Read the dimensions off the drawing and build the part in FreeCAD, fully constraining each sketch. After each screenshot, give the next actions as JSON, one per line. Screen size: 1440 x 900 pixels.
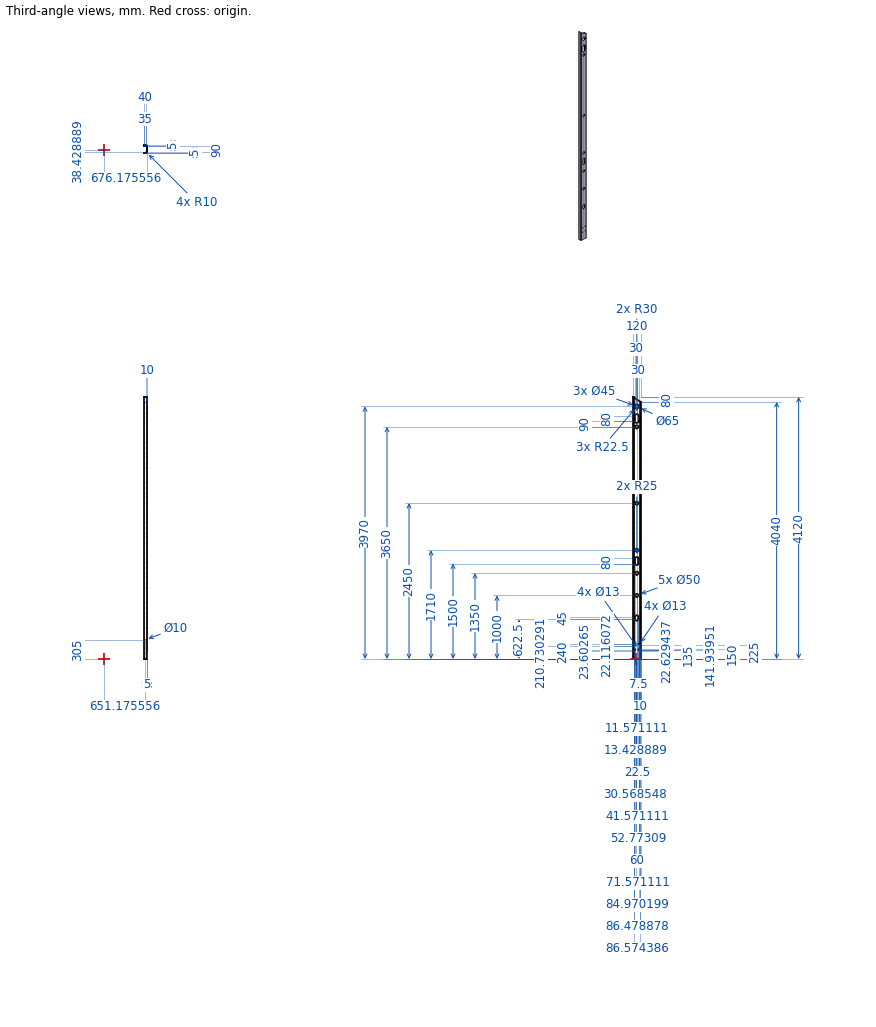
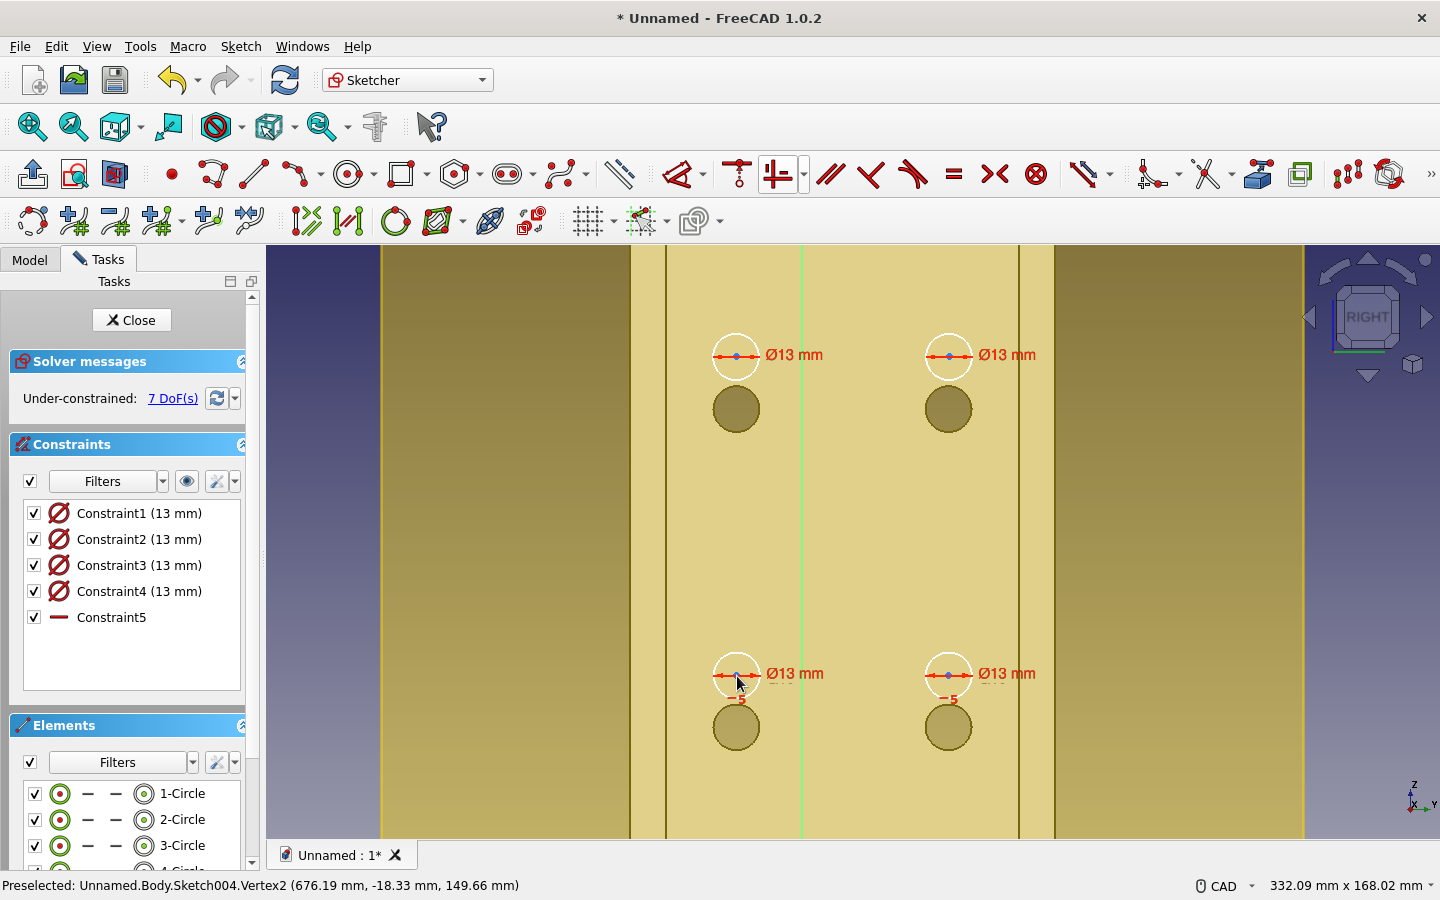
{"action": "left_click", "coordinate": [737, 676]}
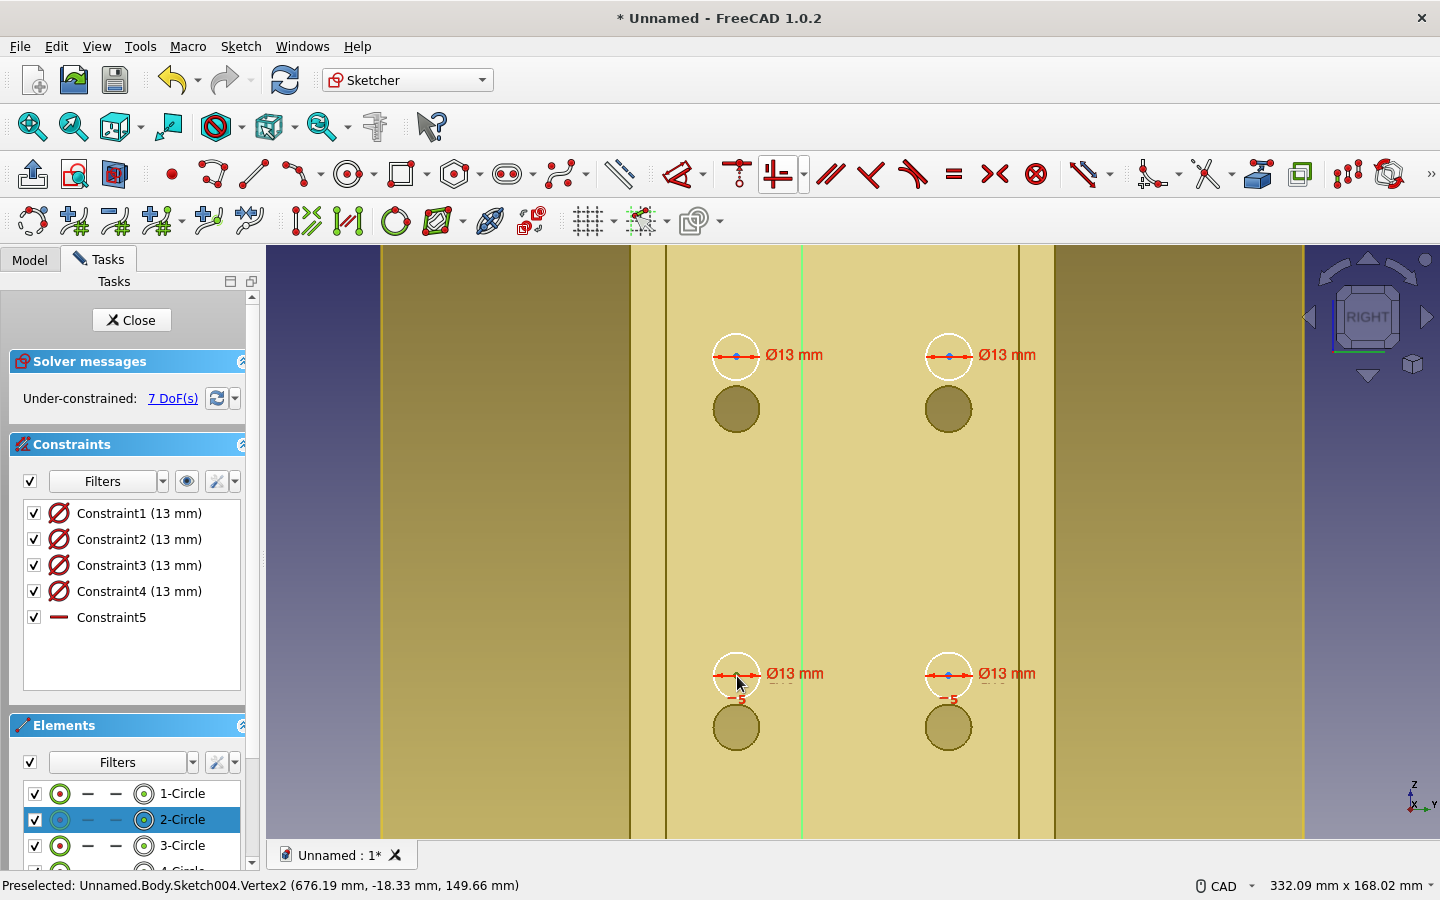
{"action": "left_click", "coordinate": [736, 357]}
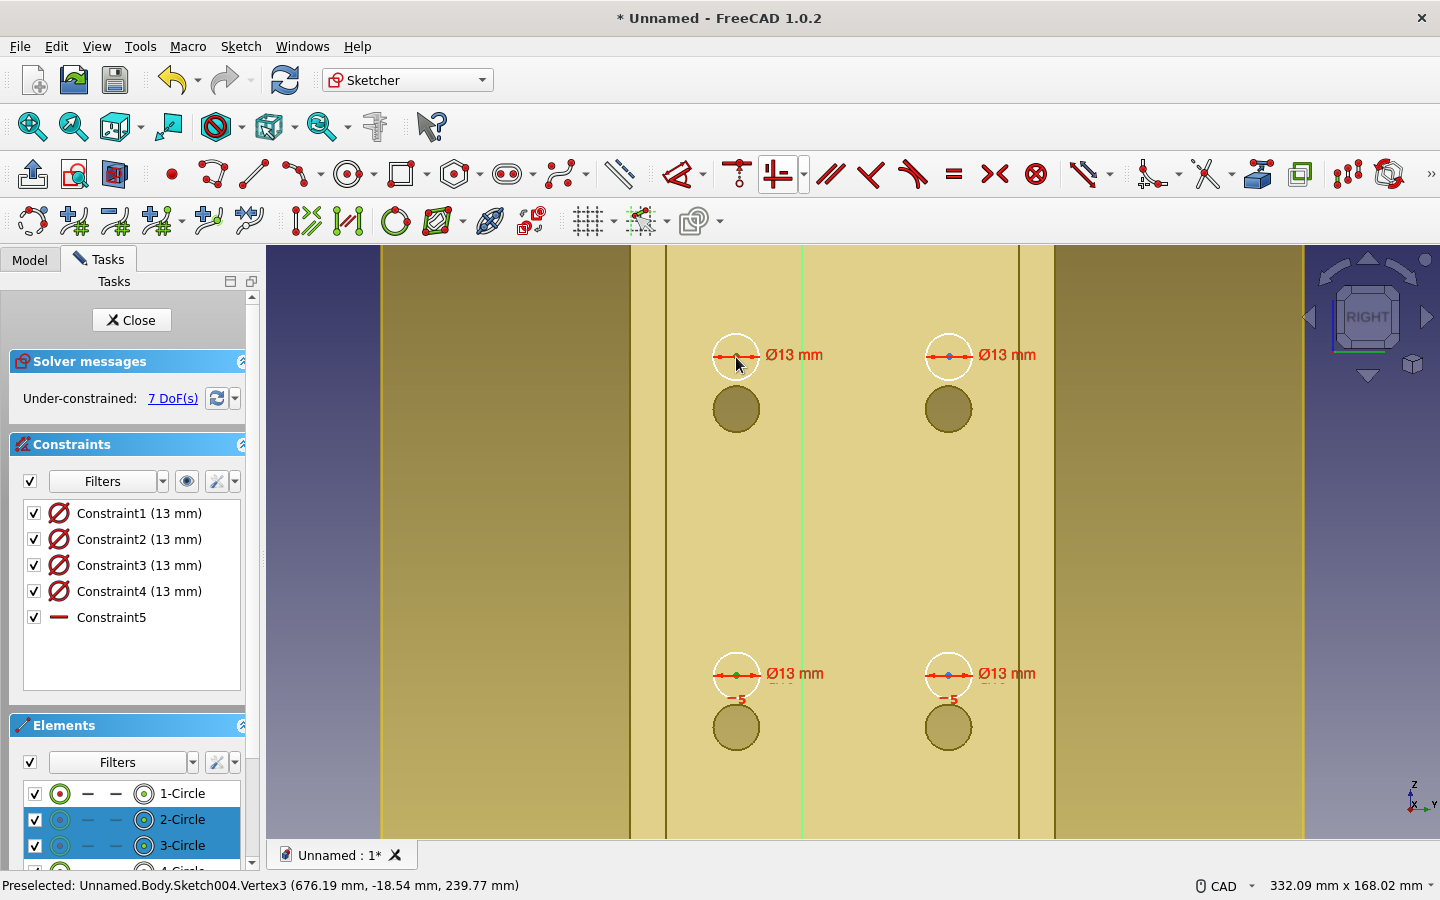
{"action": "key", "text": "v"}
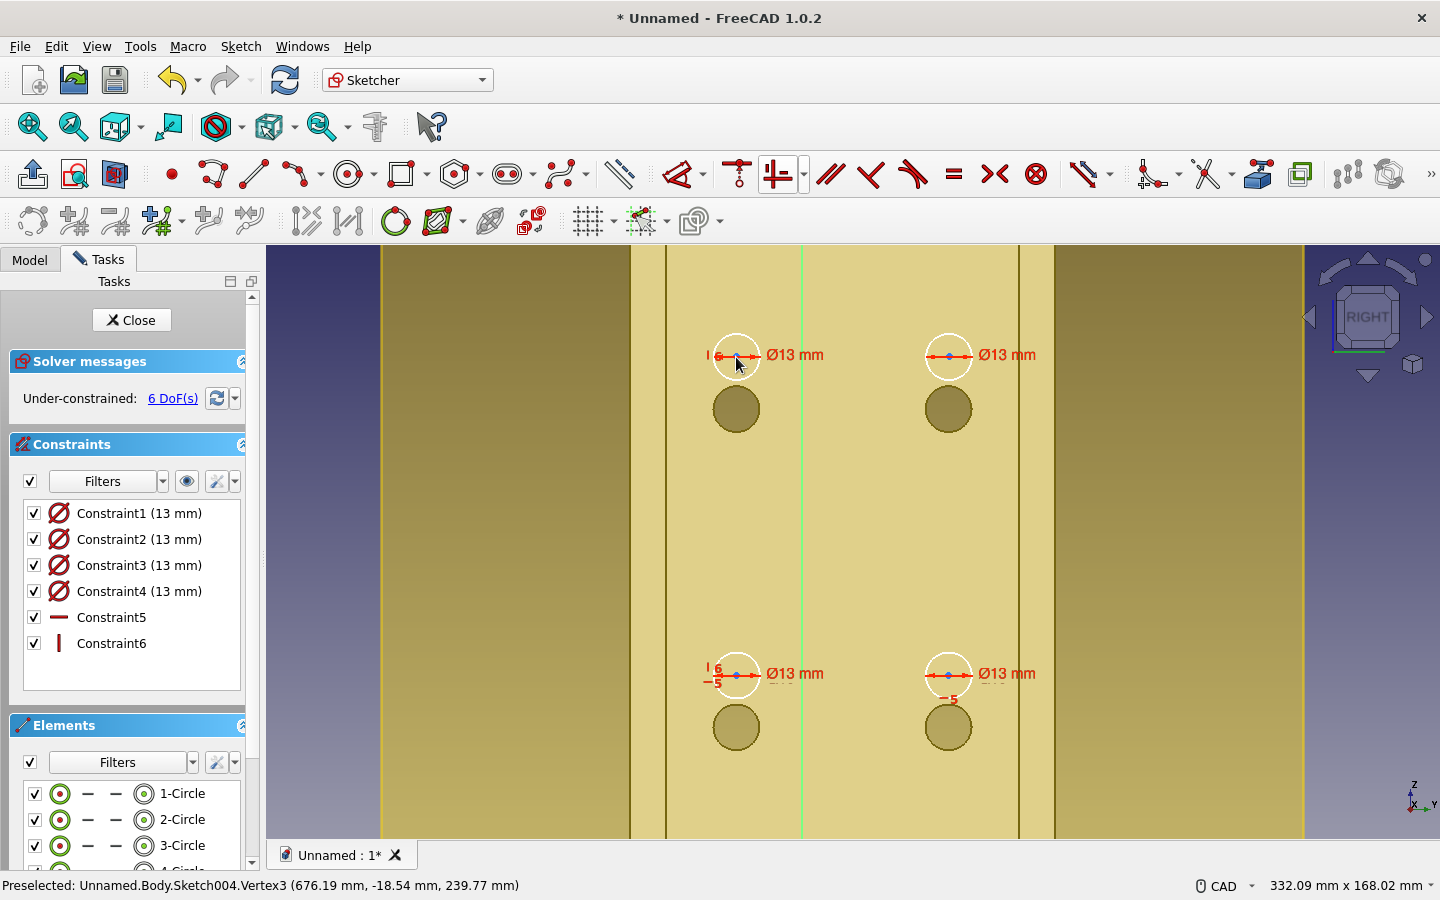
{"action": "left_click", "coordinate": [949, 676]}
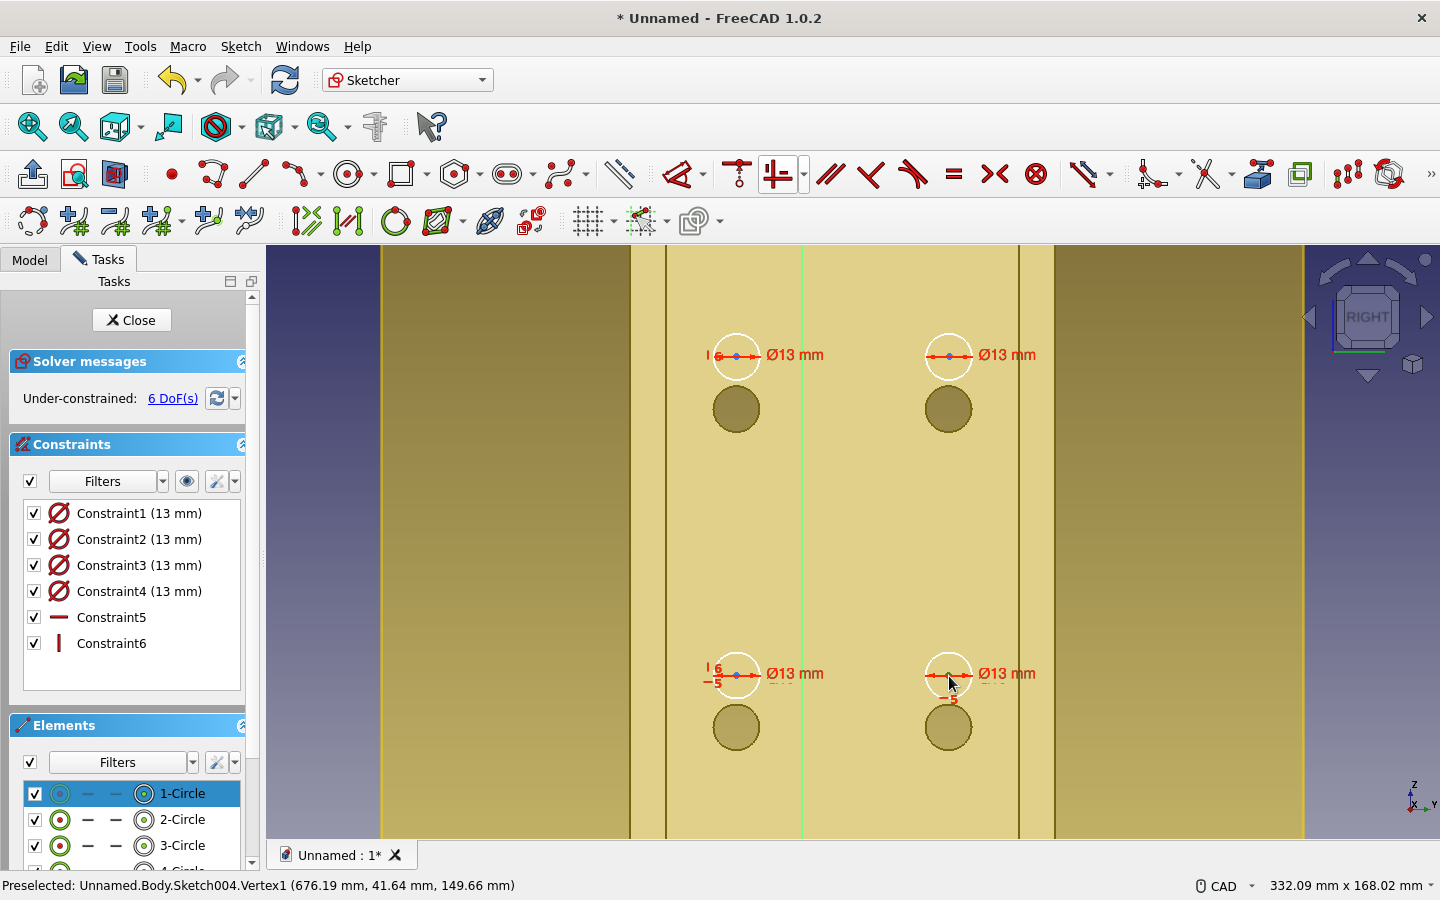
{"action": "left_click", "coordinate": [949, 357]}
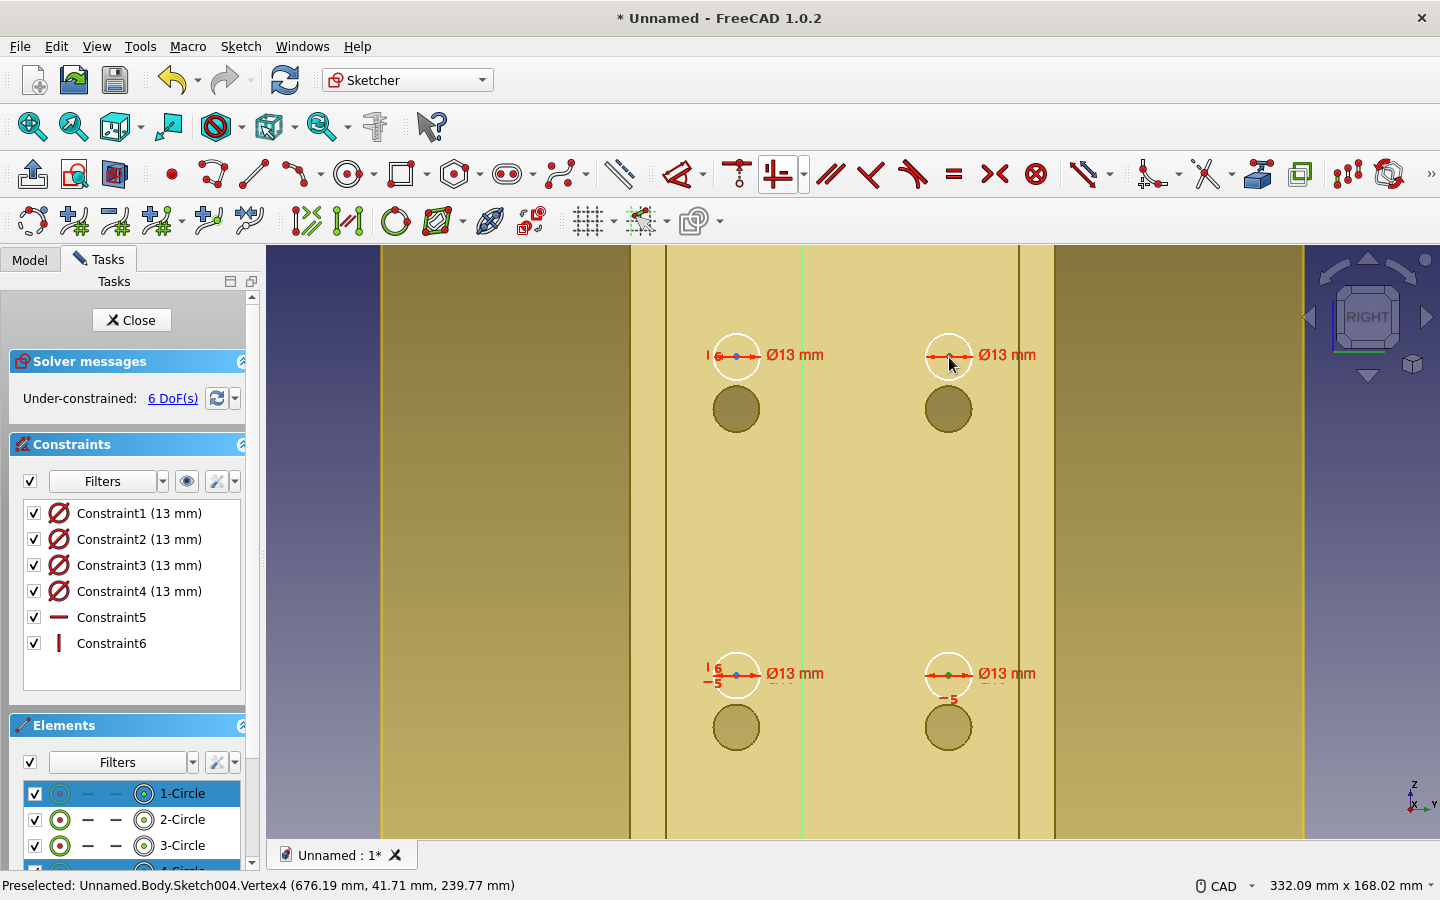
{"action": "key", "text": "v"}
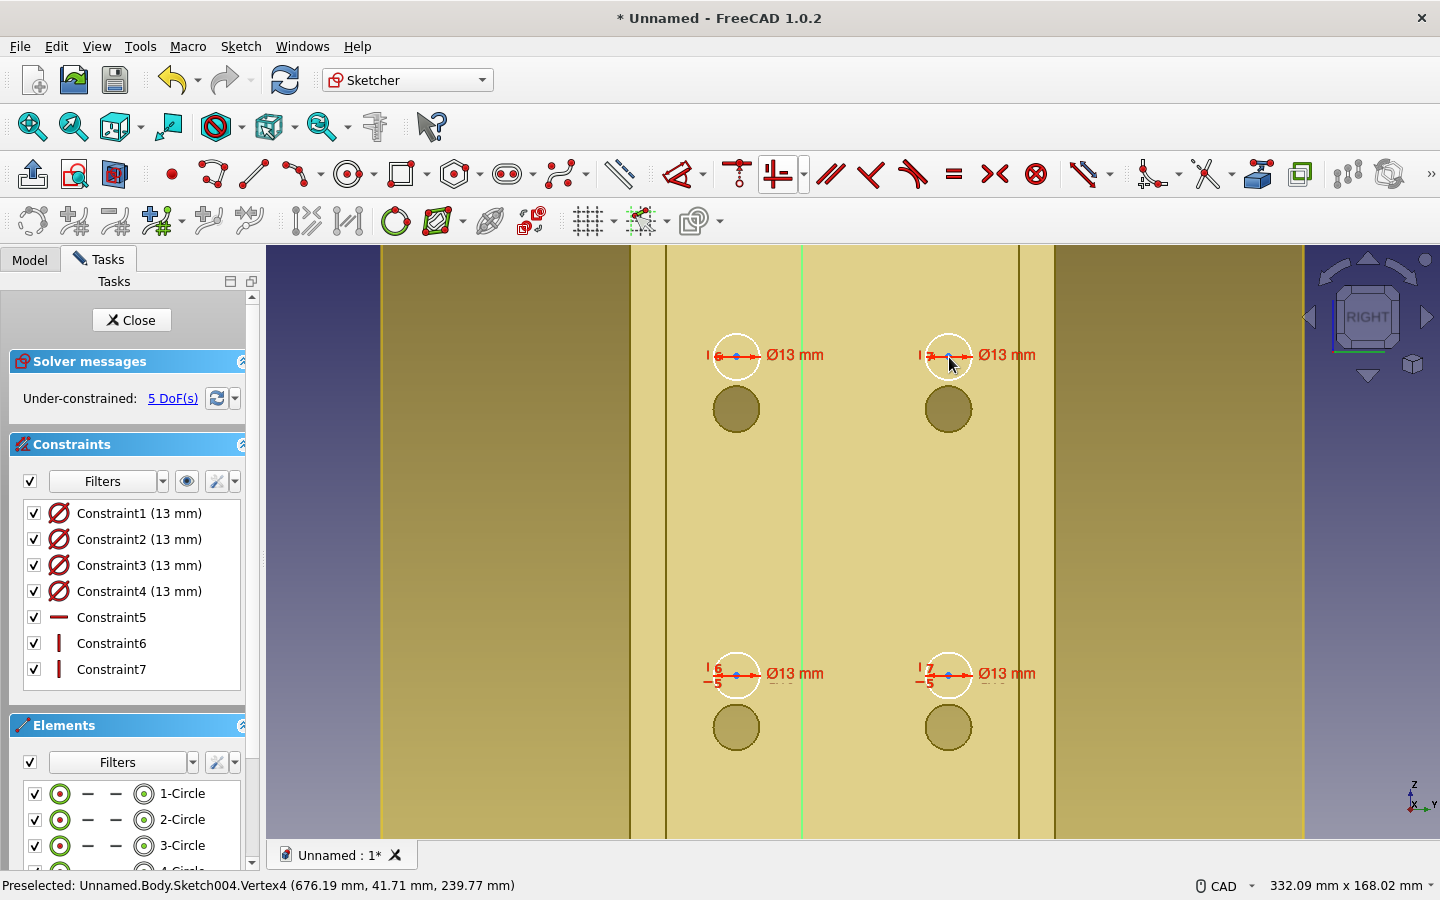
{"action": "left_click", "coordinate": [737, 357]}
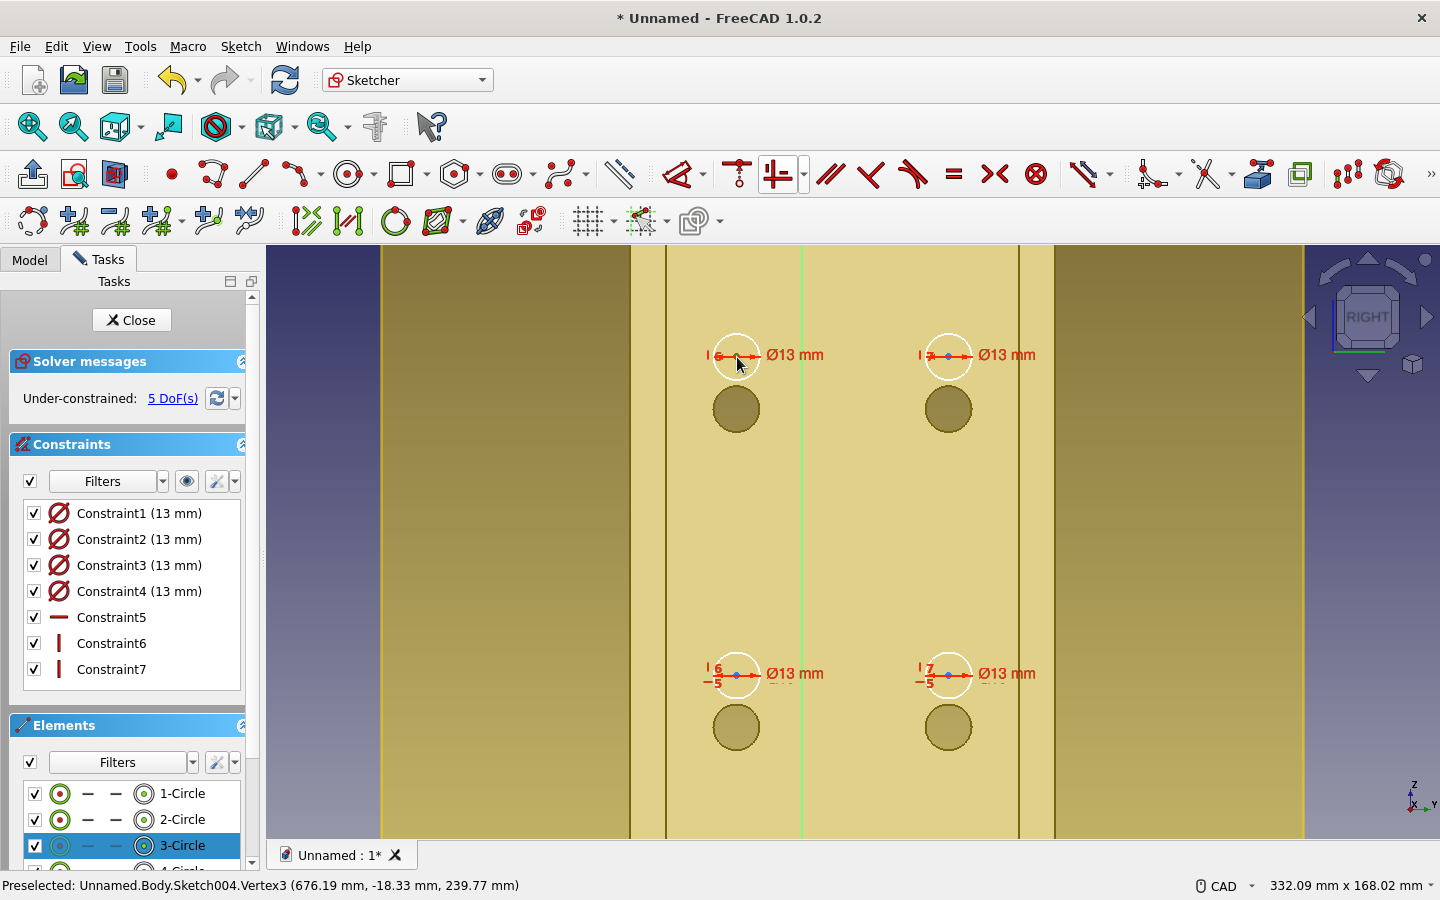
{"action": "left_click", "coordinate": [949, 357]}